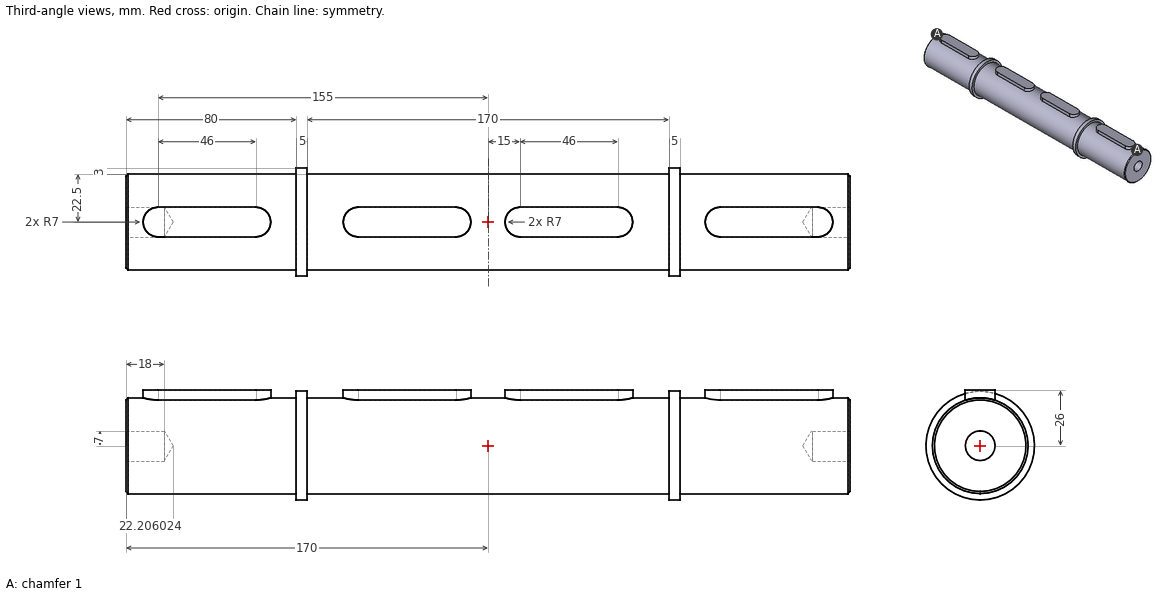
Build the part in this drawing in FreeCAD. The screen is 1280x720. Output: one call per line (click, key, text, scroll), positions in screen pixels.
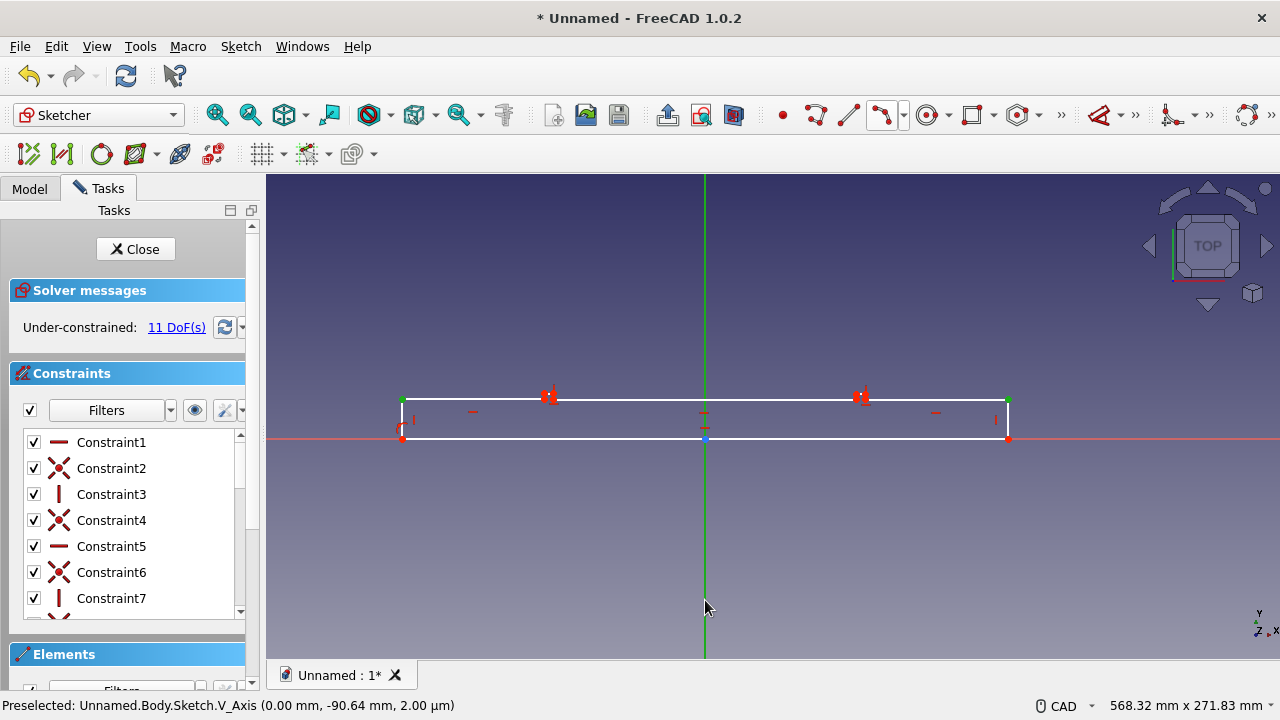
key(s)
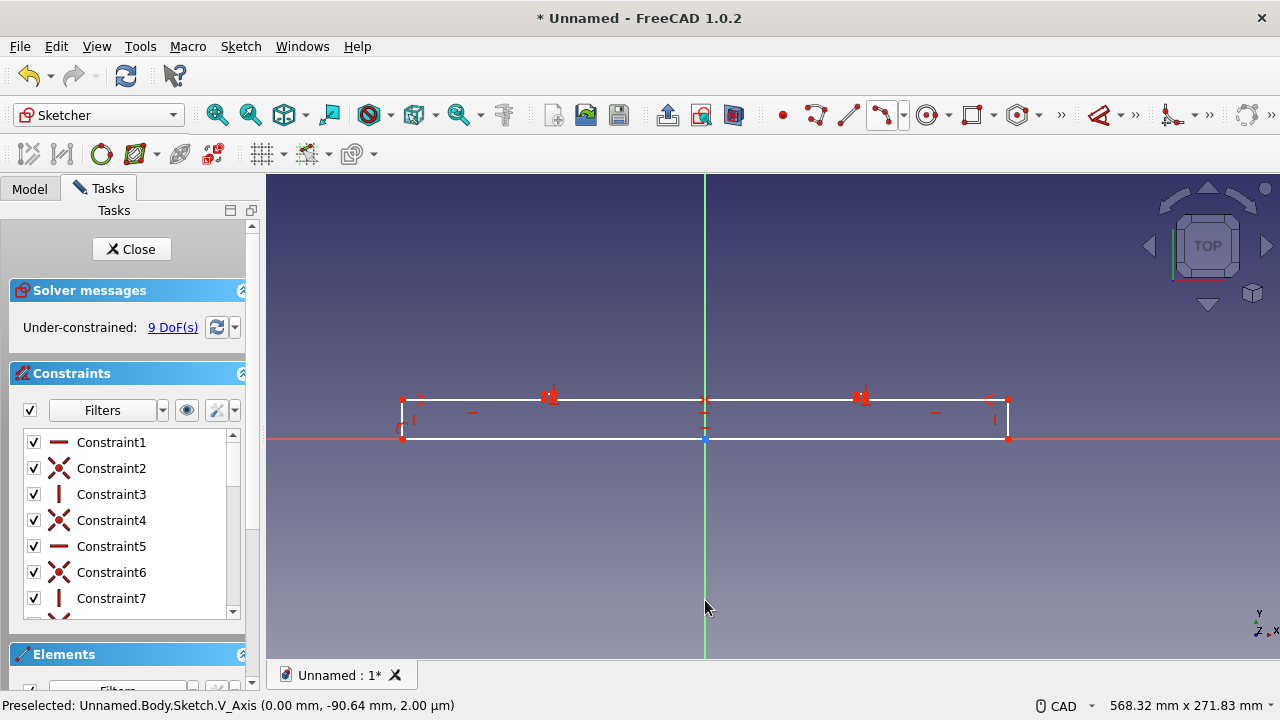
scroll(545, 394, up, 4)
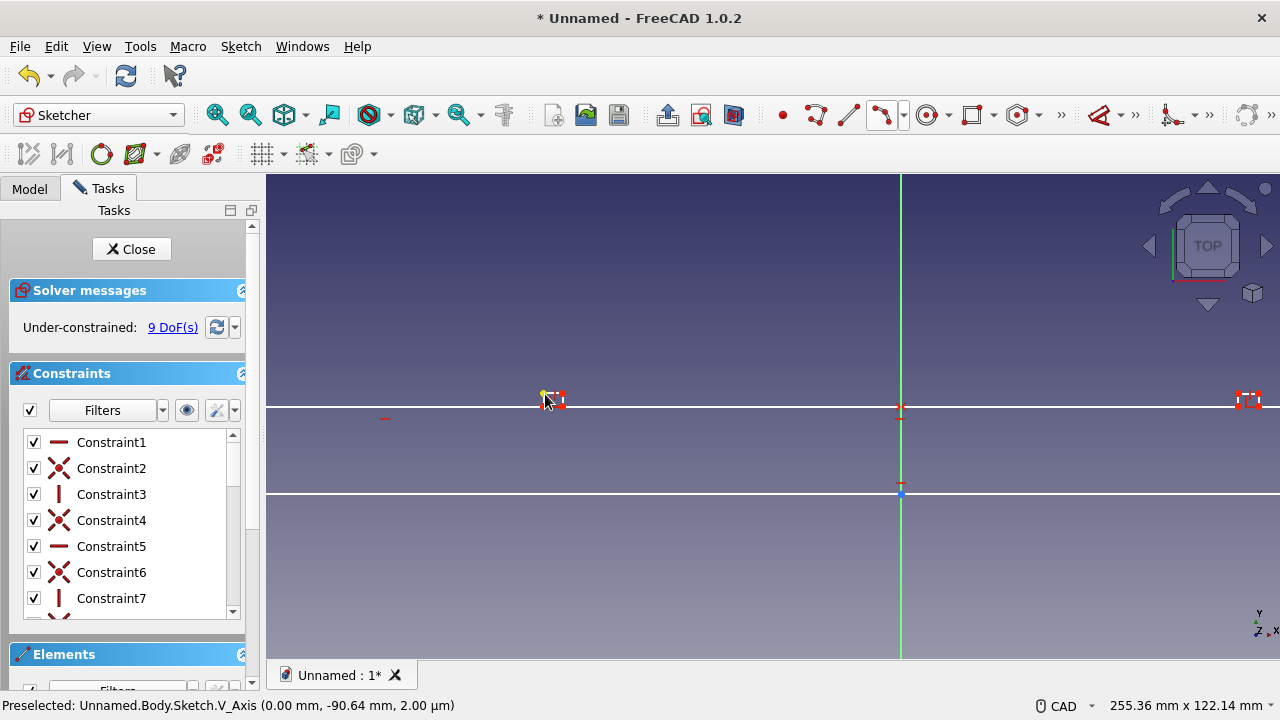
click(544, 393)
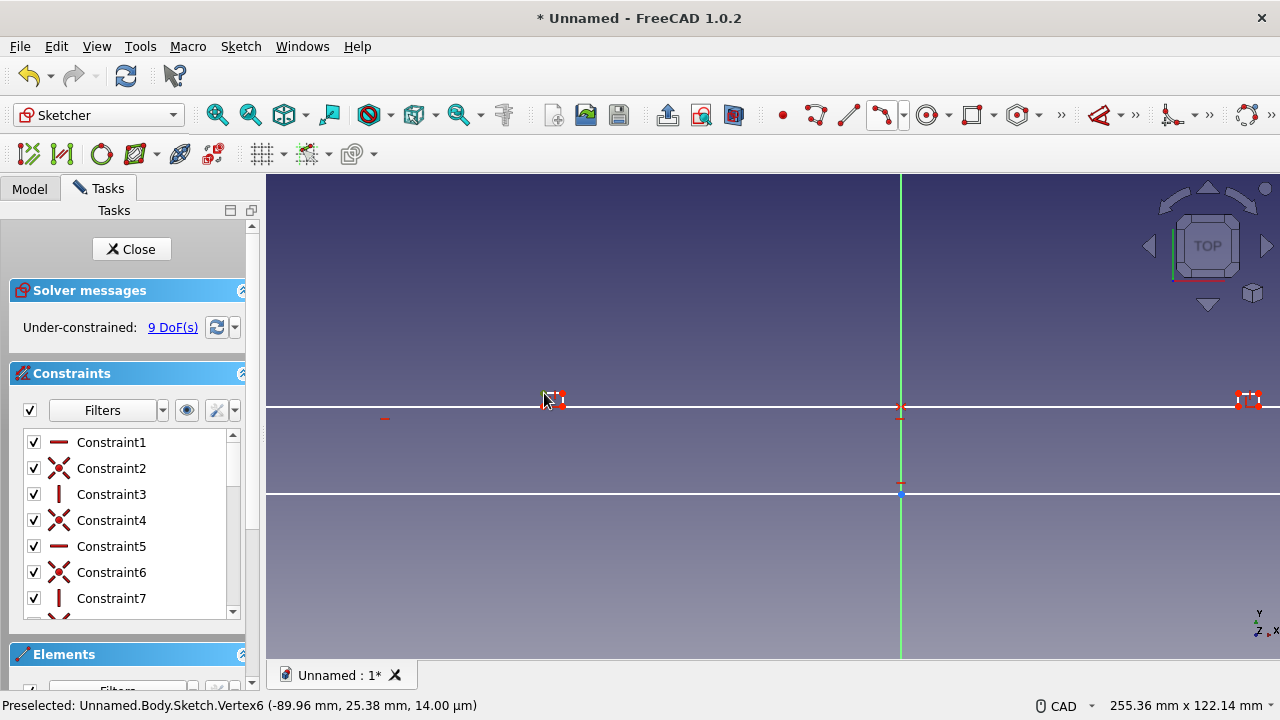
scroll(544, 394, down, 4)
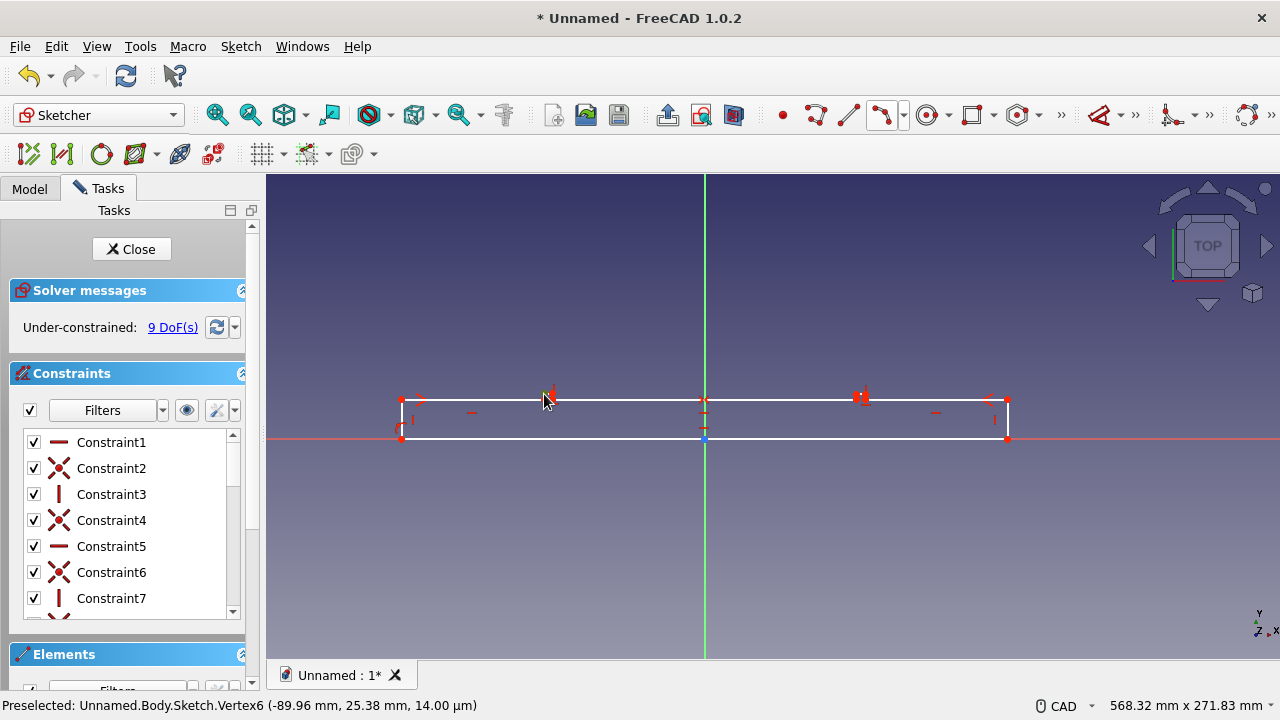
scroll(865, 394, up, 4)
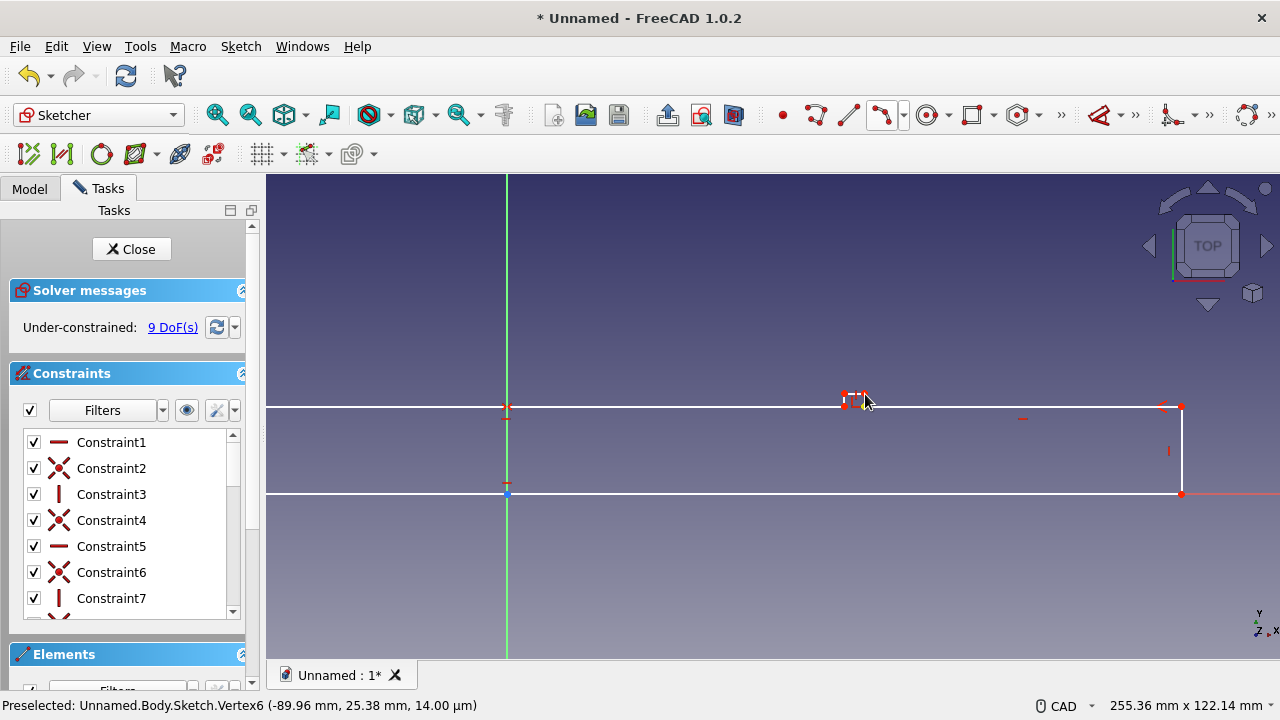
click(865, 394)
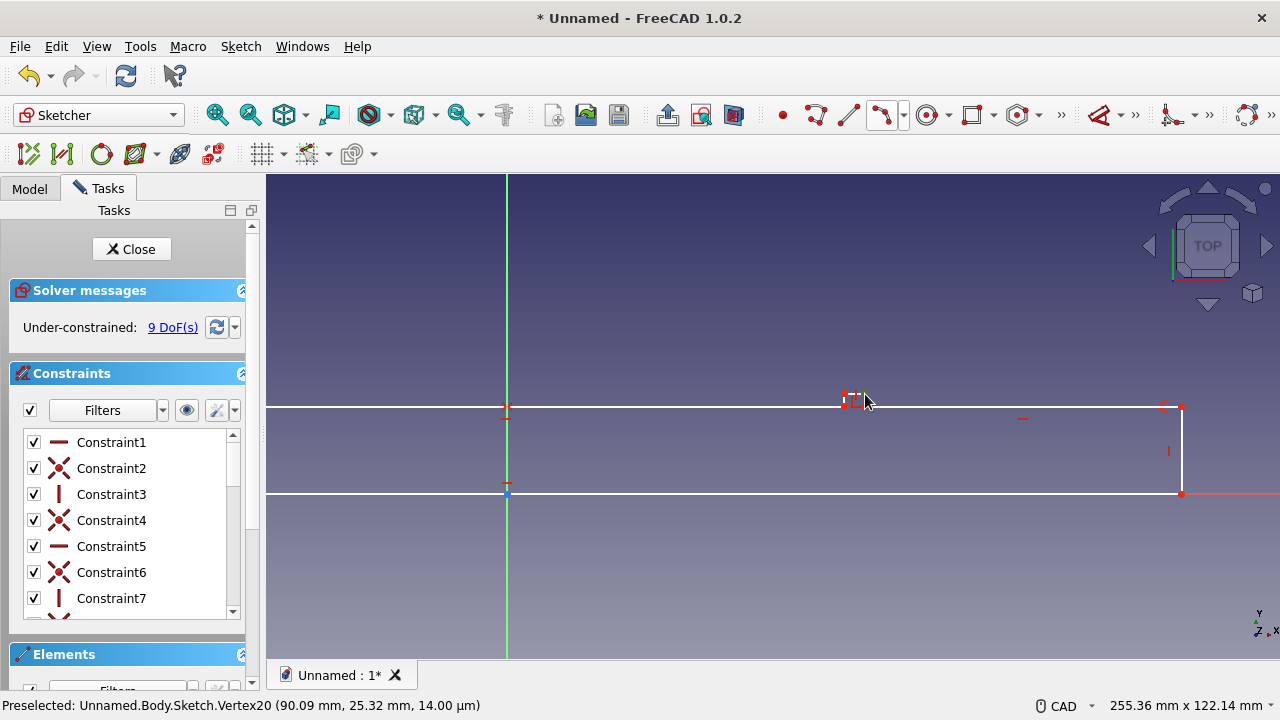
click(507, 600)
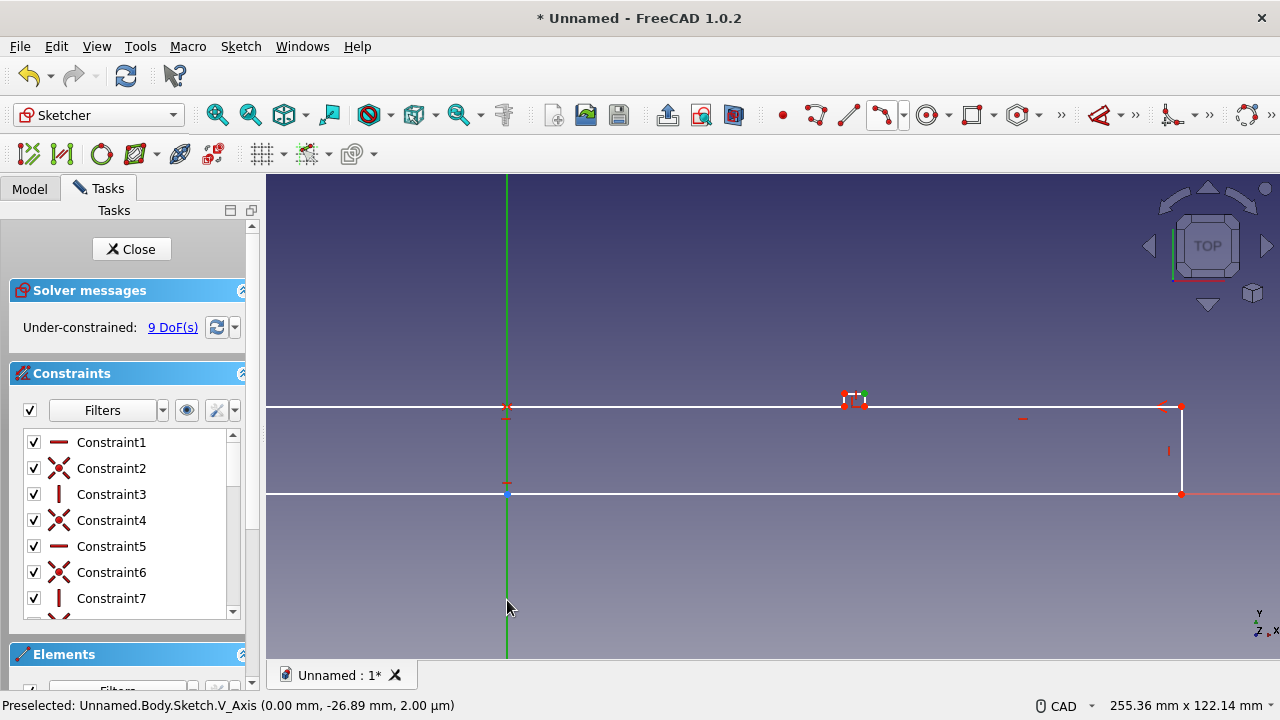
key(s)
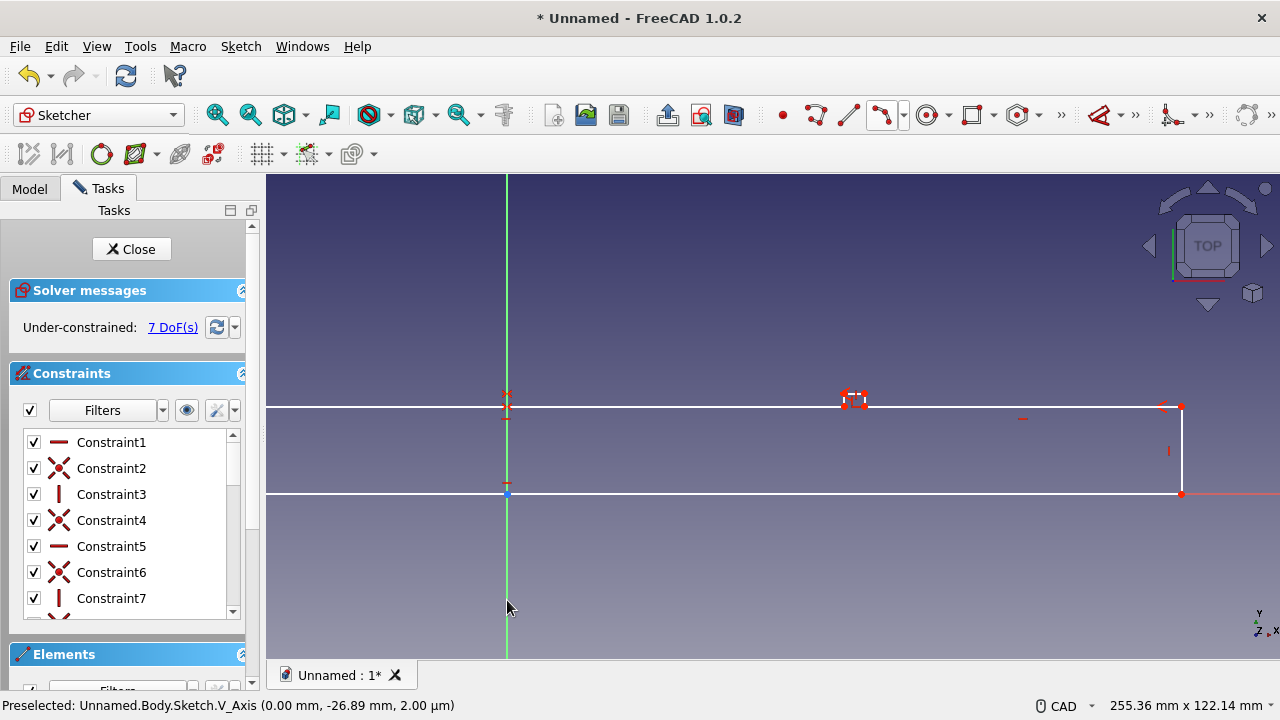
click(1098, 116)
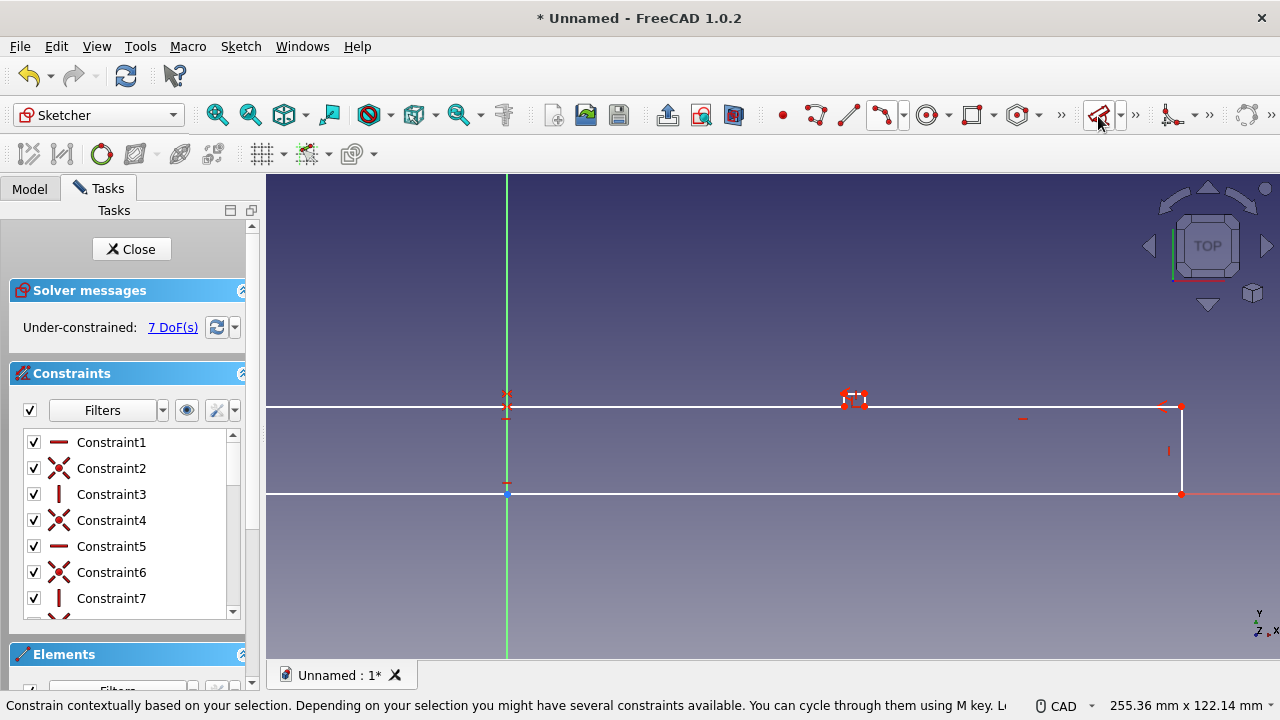
scroll(865, 394, down, 4)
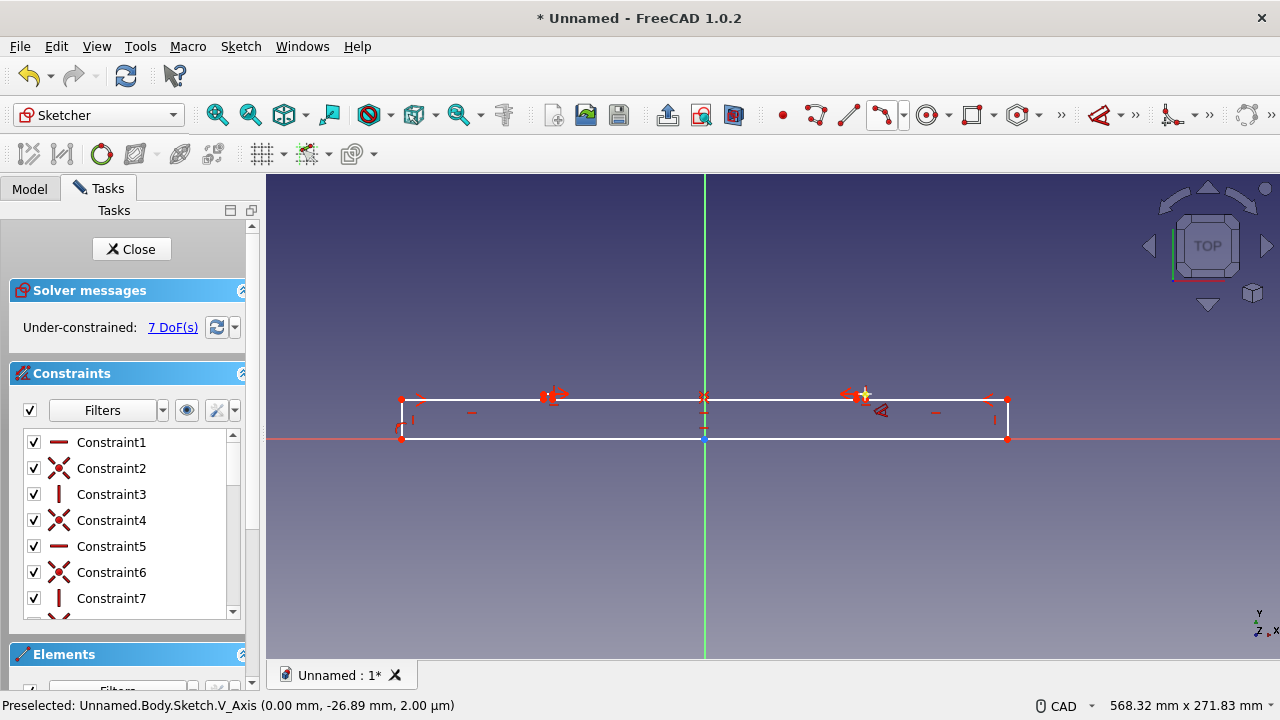
scroll(553, 397, up, 11)